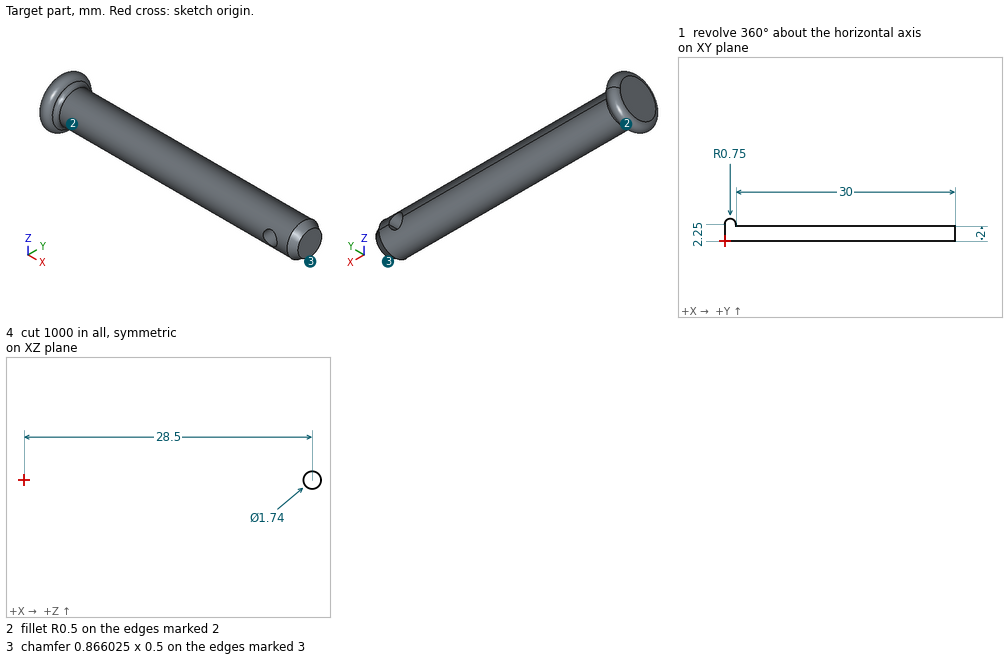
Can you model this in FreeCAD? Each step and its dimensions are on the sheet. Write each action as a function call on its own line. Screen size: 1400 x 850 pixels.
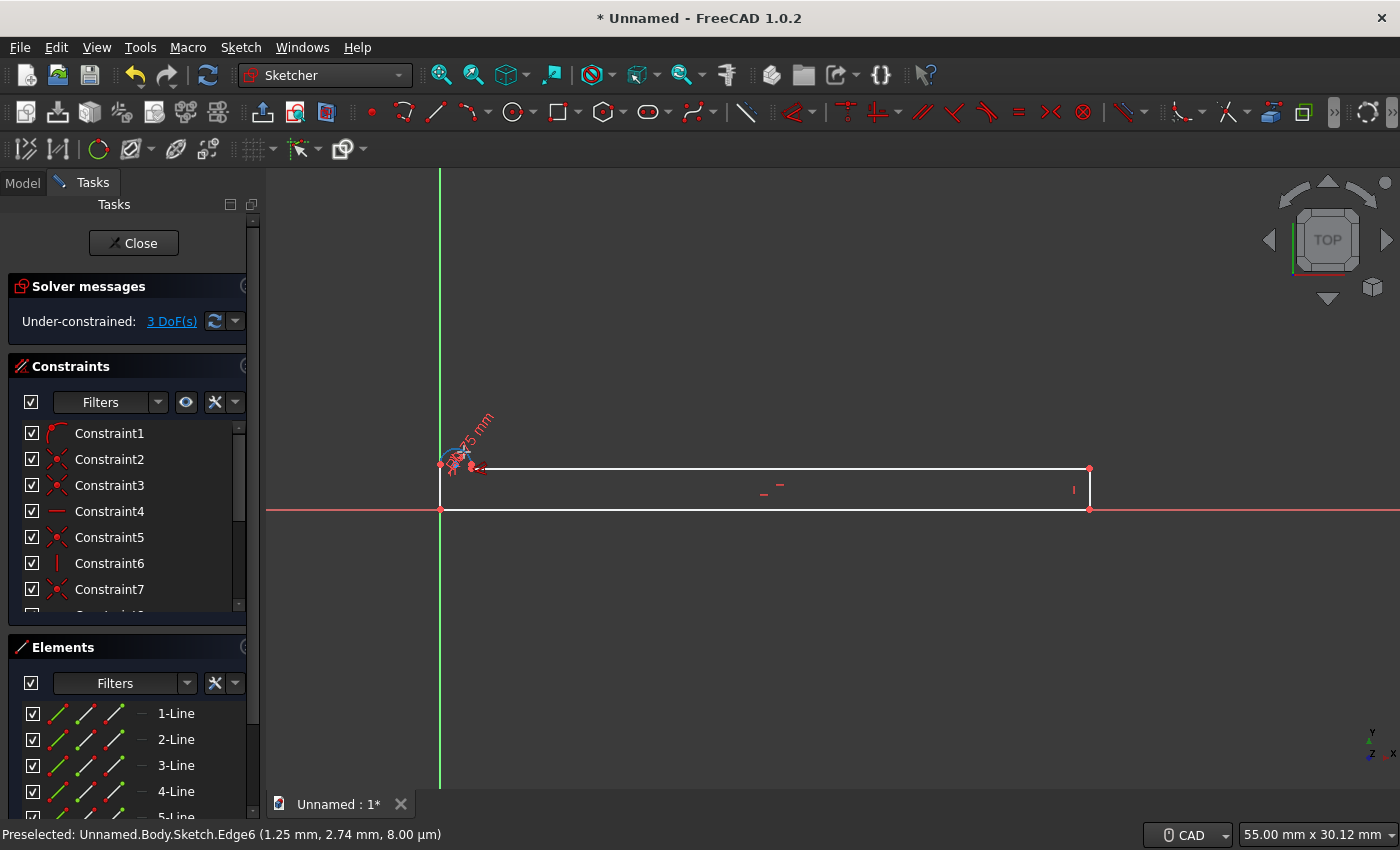
click(1090, 497)
click(1124, 489)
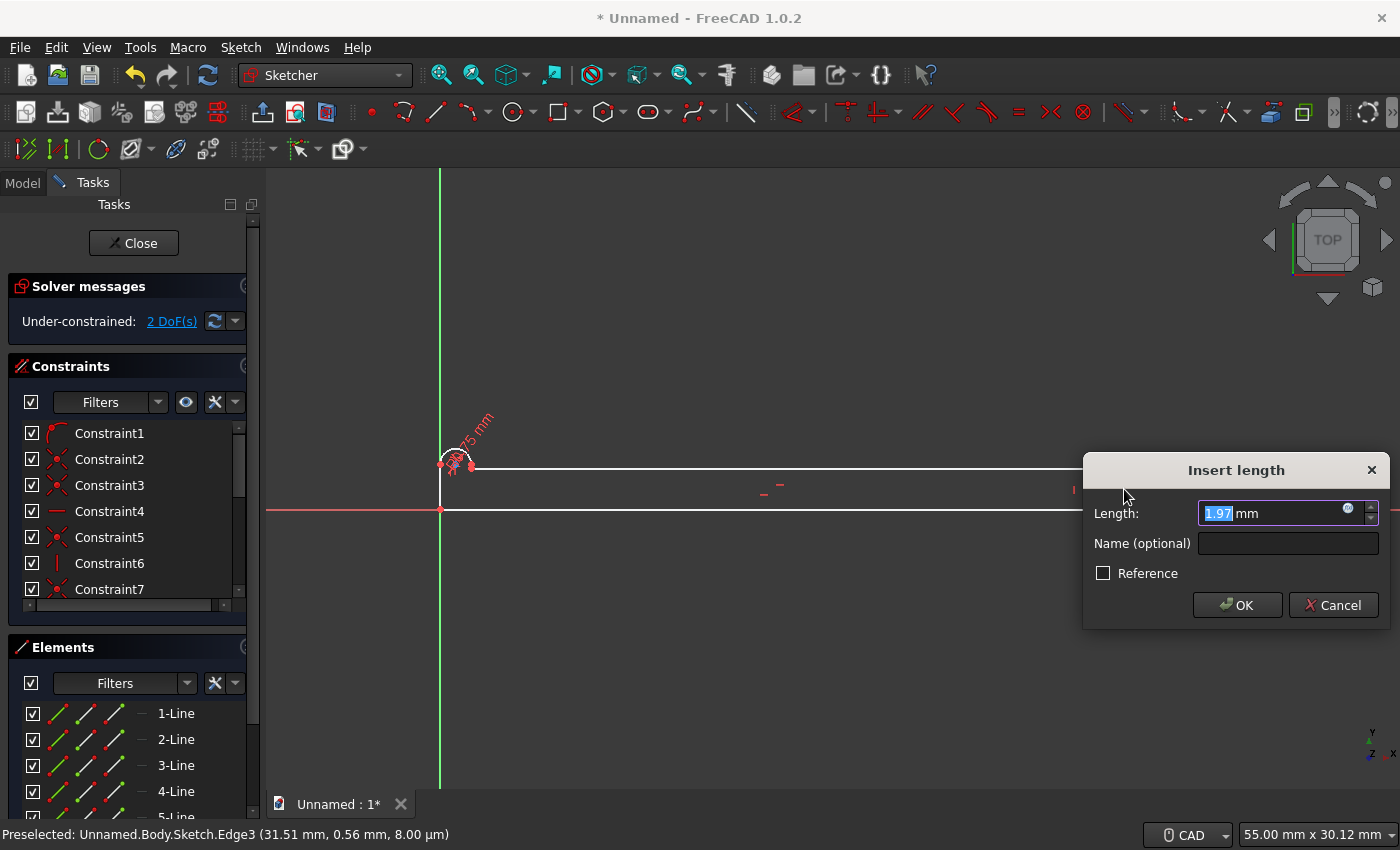
text(2)
key(Return)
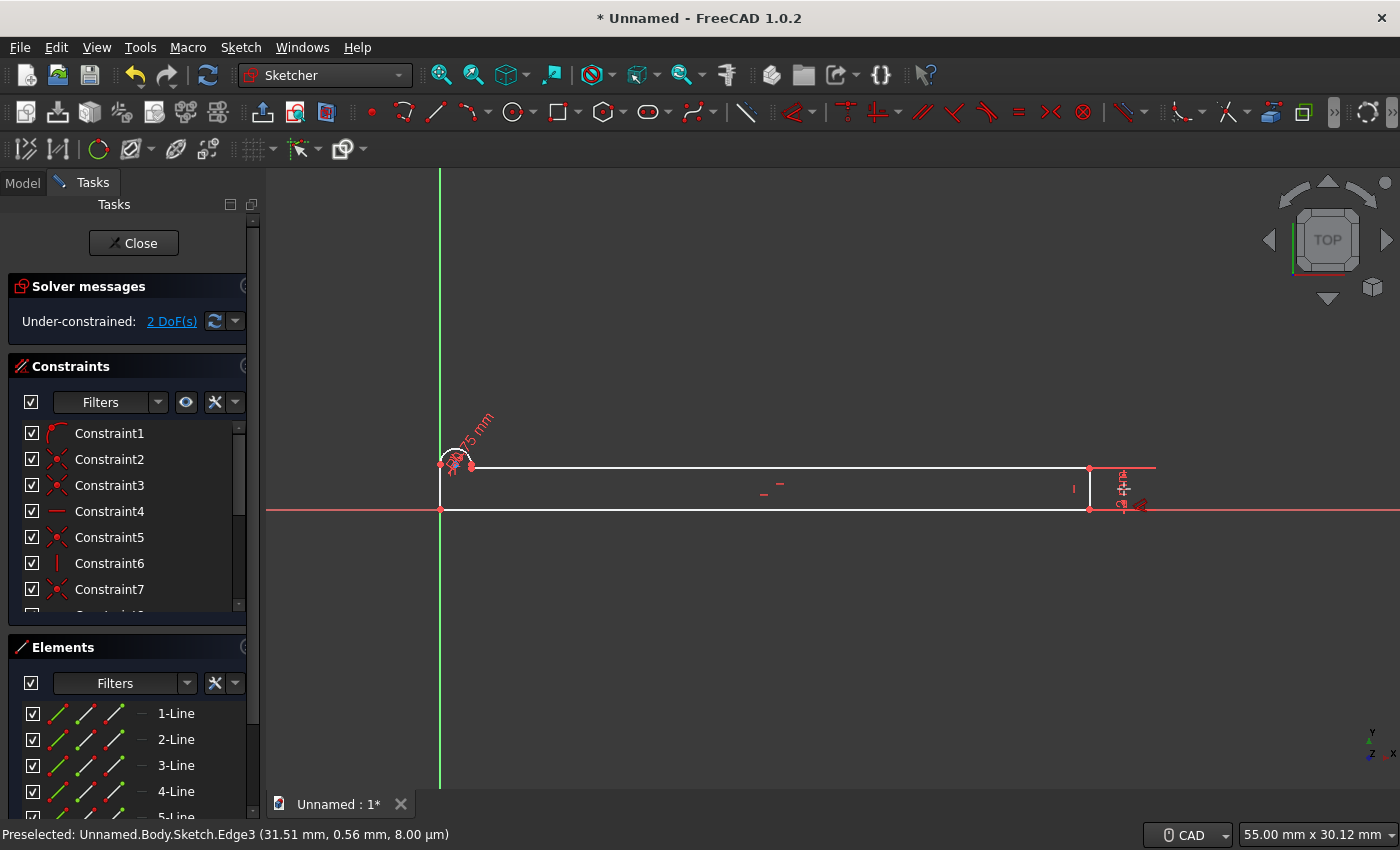
click(904, 468)
click(780, 434)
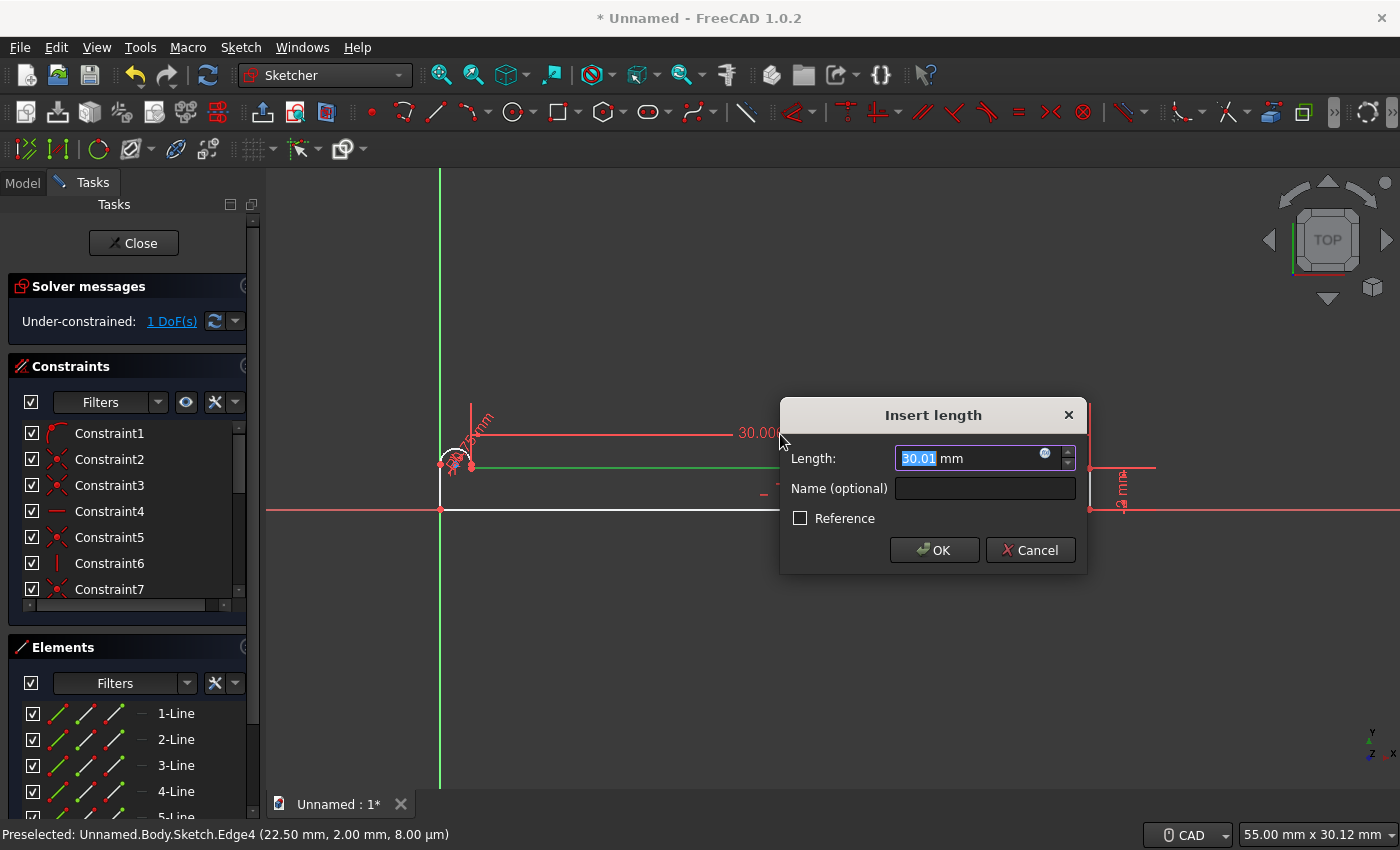
text(30)
key(Return)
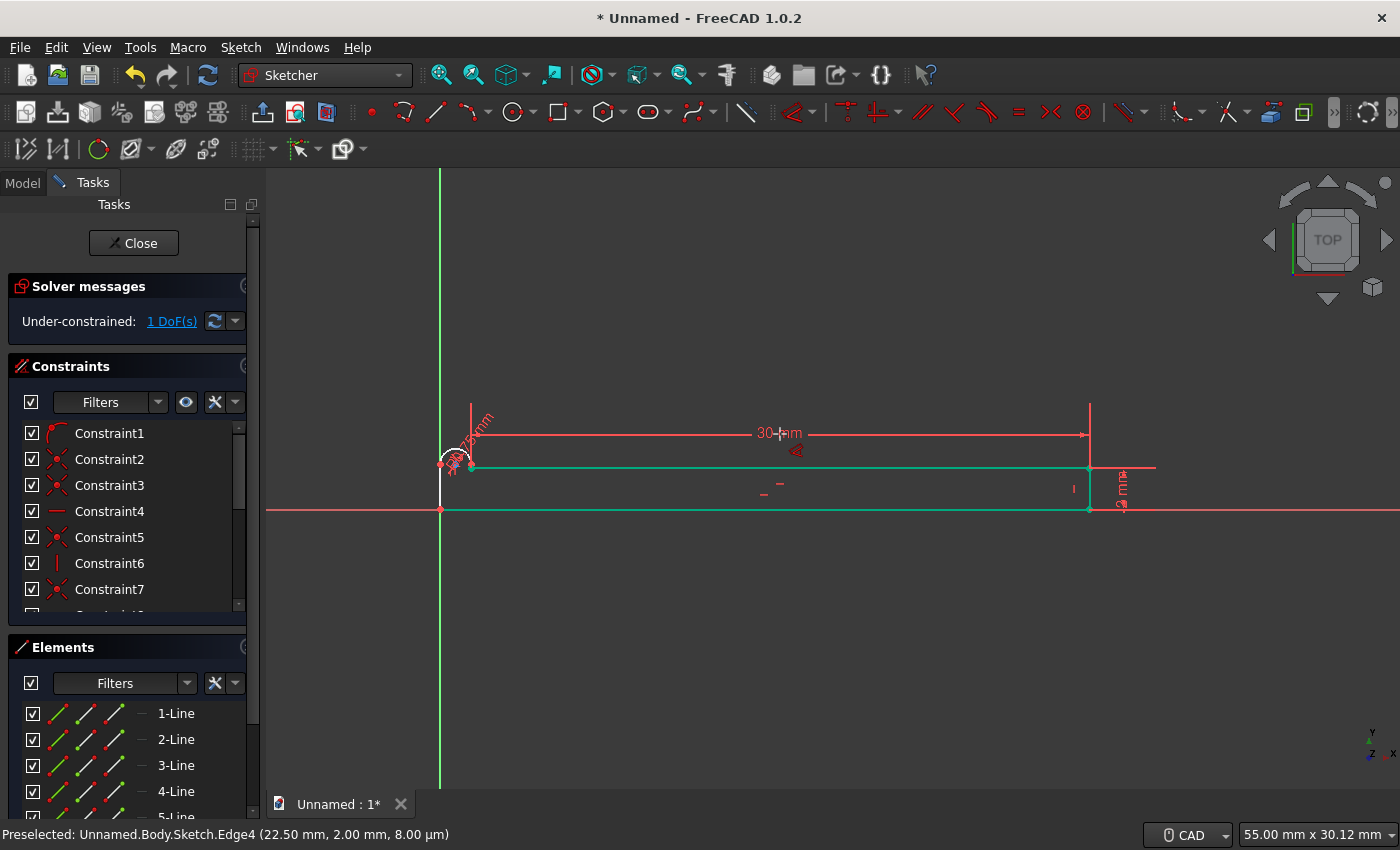
click(440, 478)
click(406, 487)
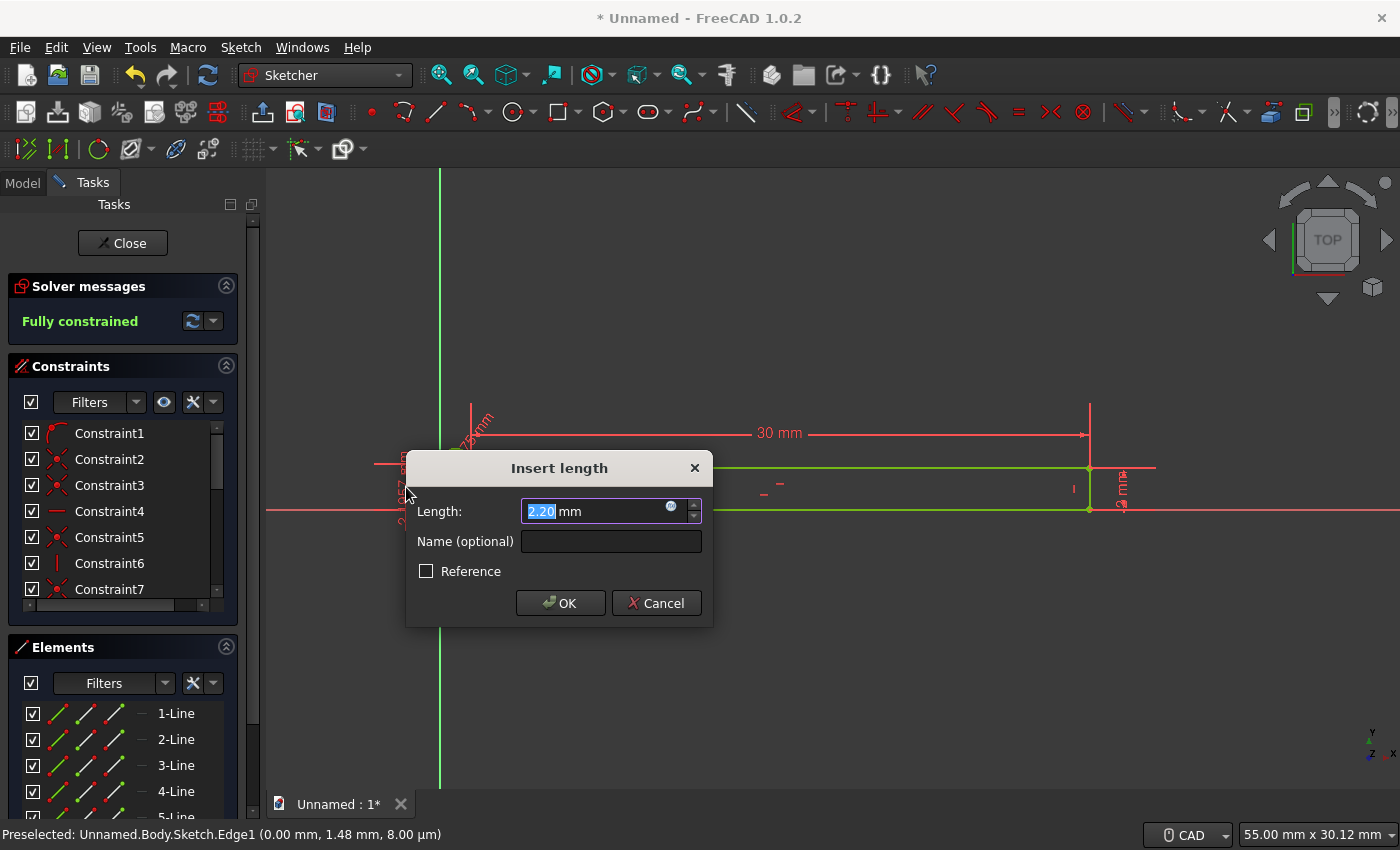
text(2.25)
key(Return)
key(Escape)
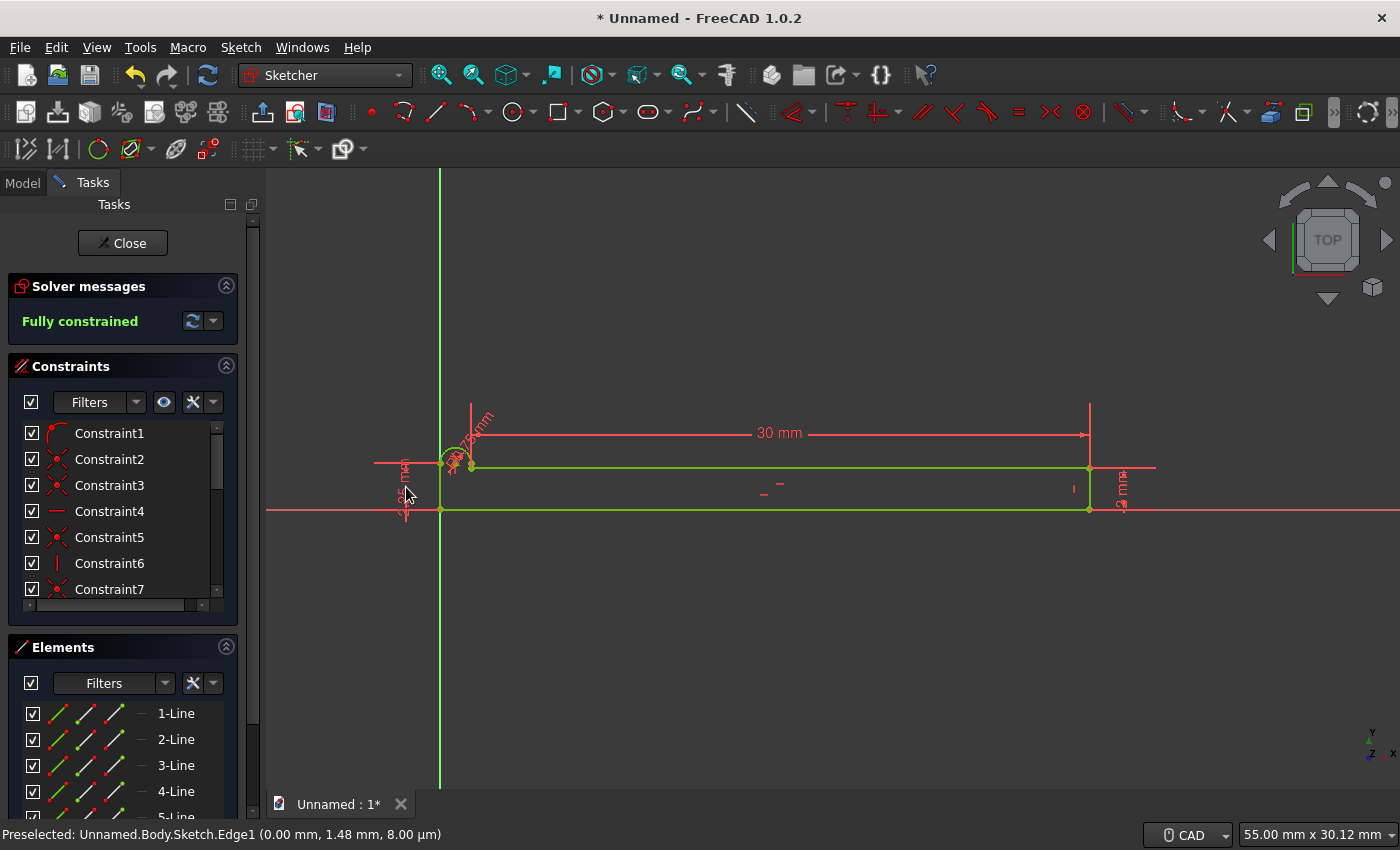
click(123, 243)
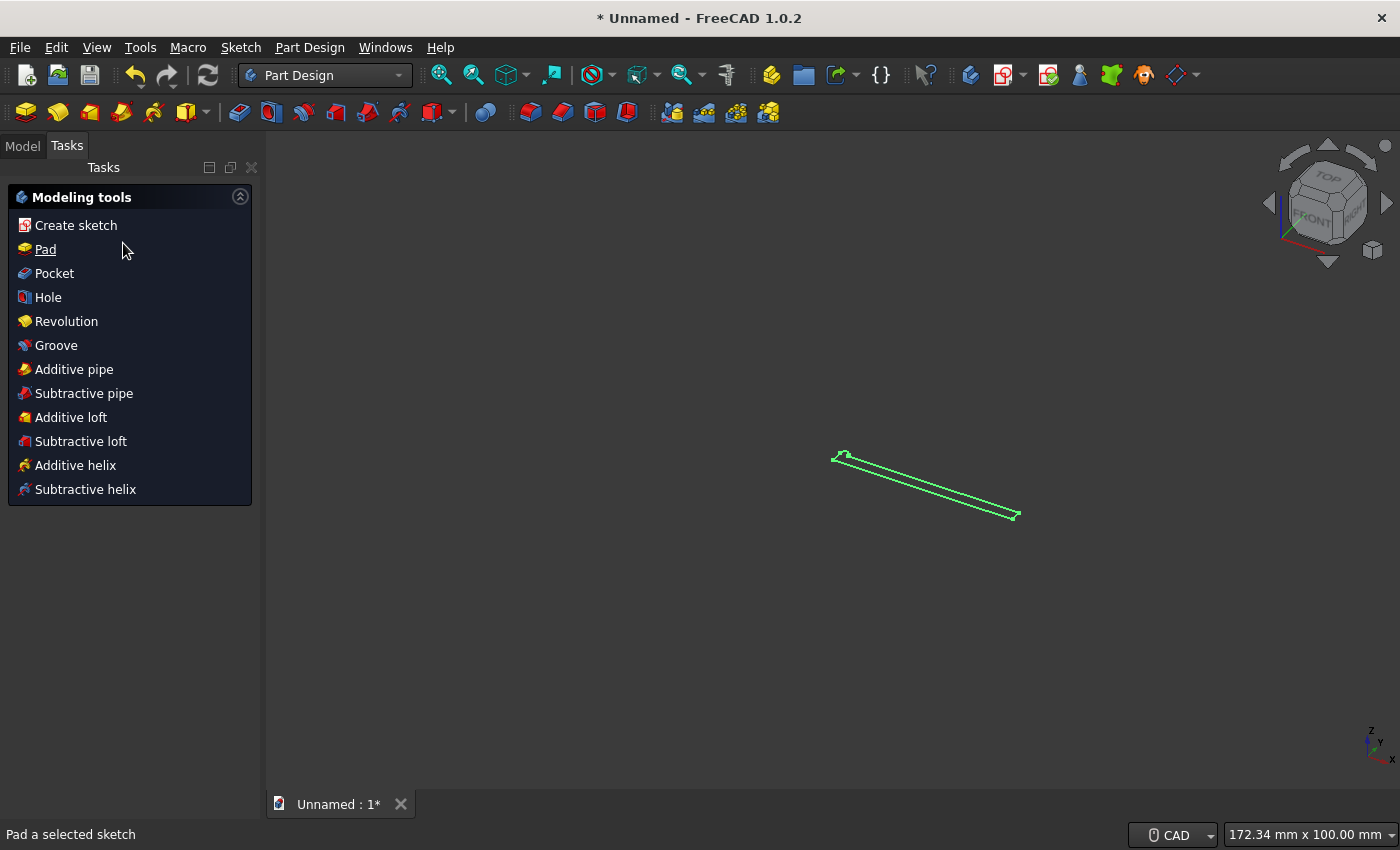
click(58, 112)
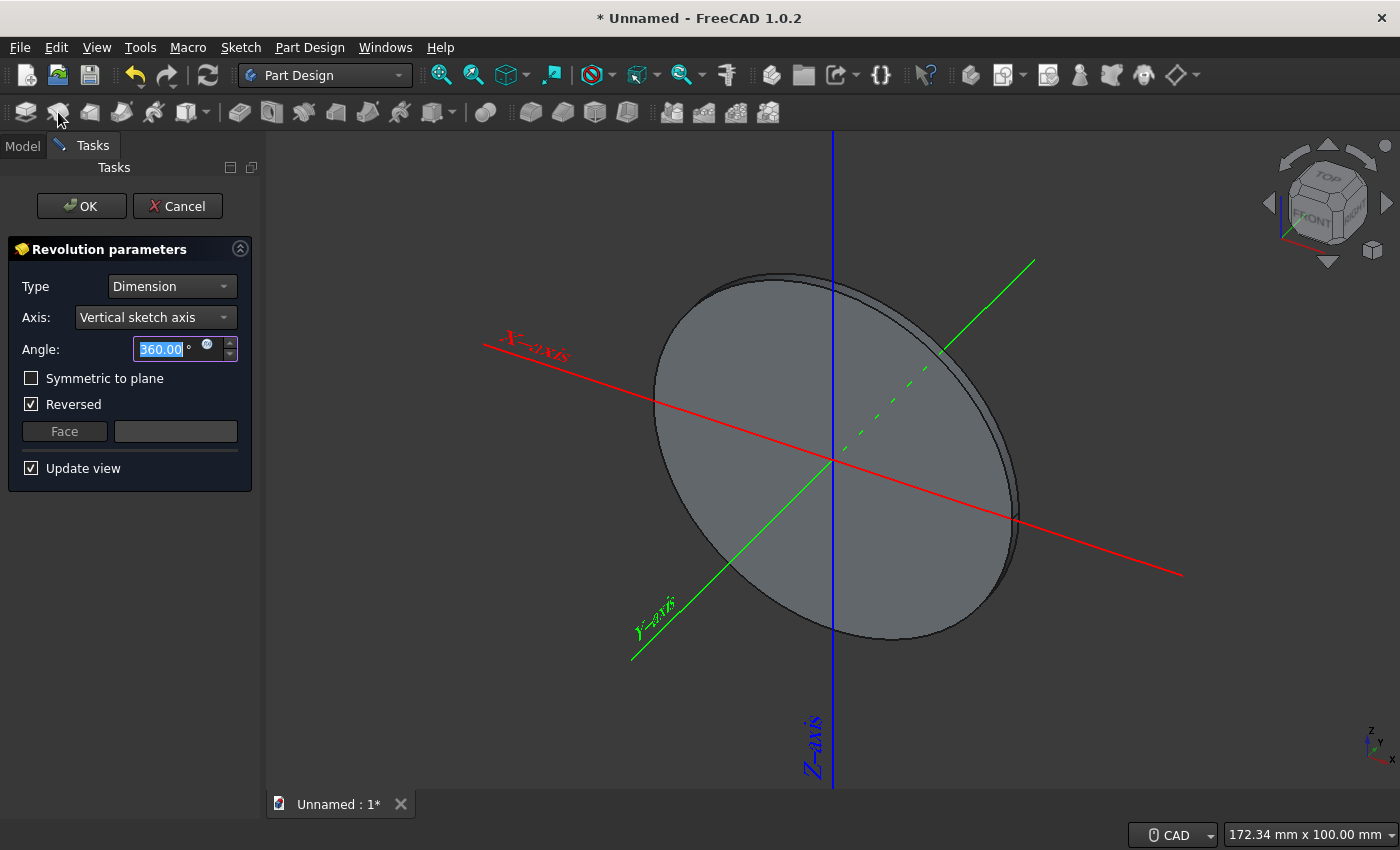
click(156, 318)